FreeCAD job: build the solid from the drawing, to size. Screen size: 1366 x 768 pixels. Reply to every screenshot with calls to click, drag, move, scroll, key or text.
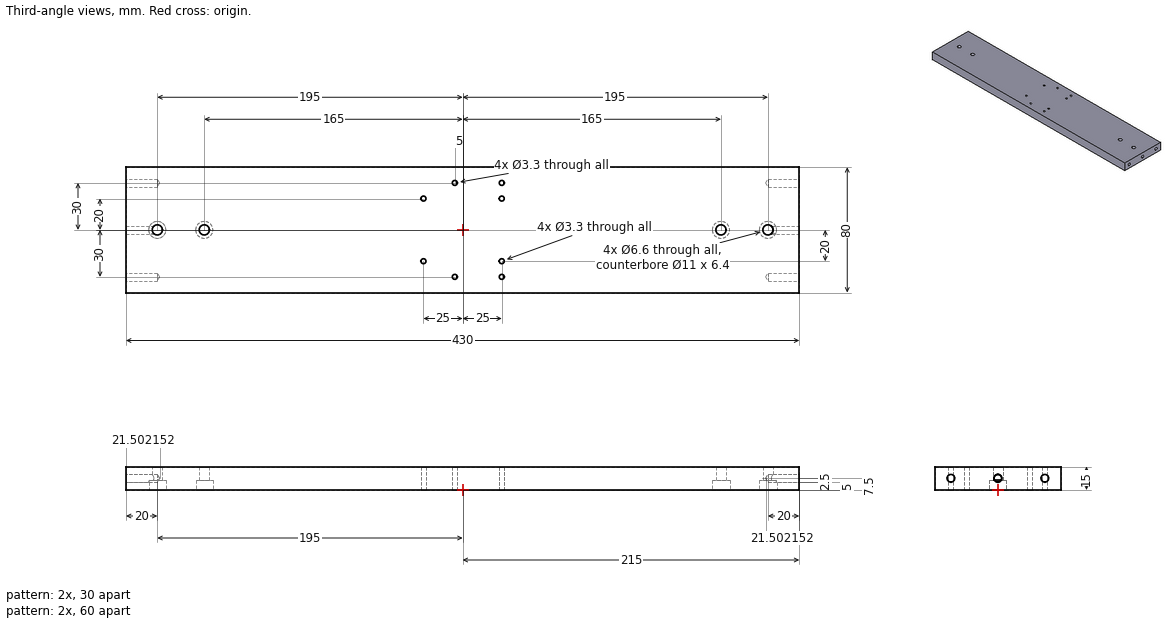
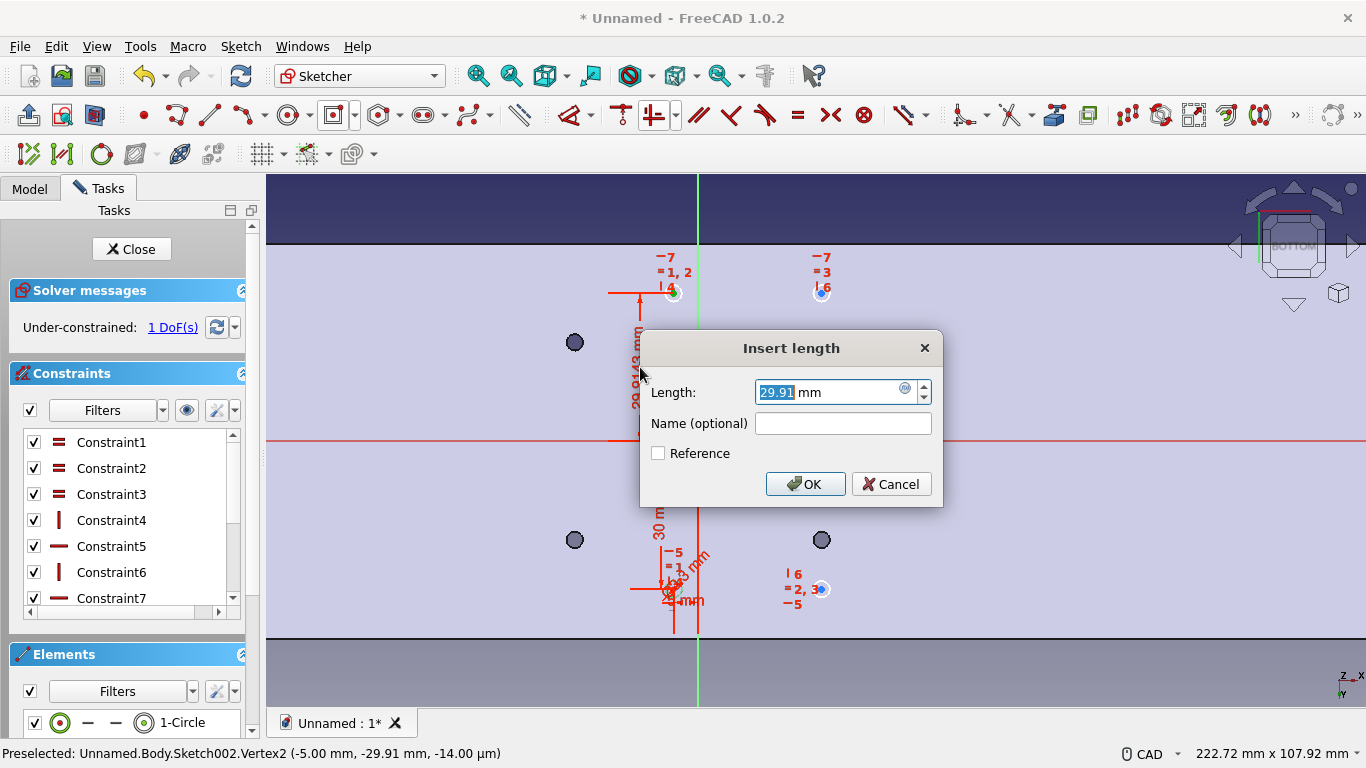
text(30)
key(Return)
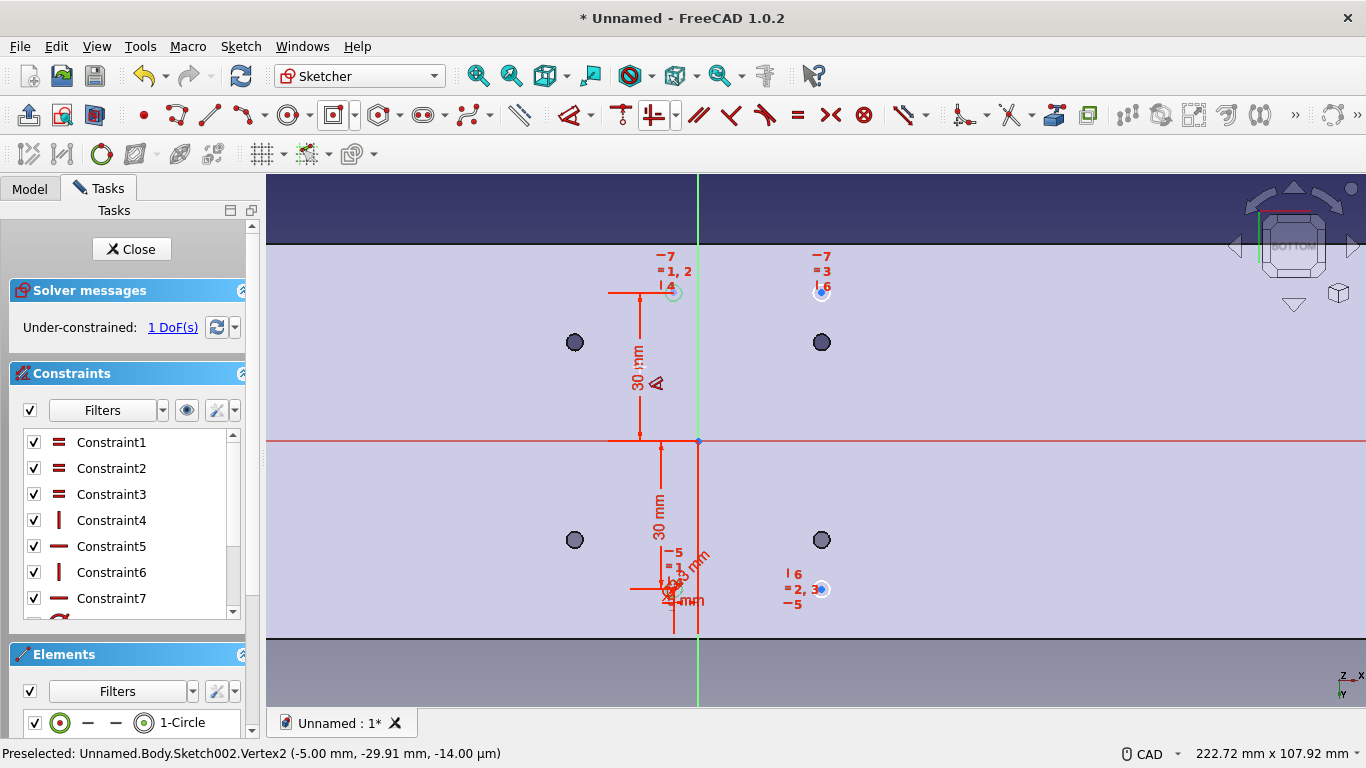
click(822, 589)
click(760, 623)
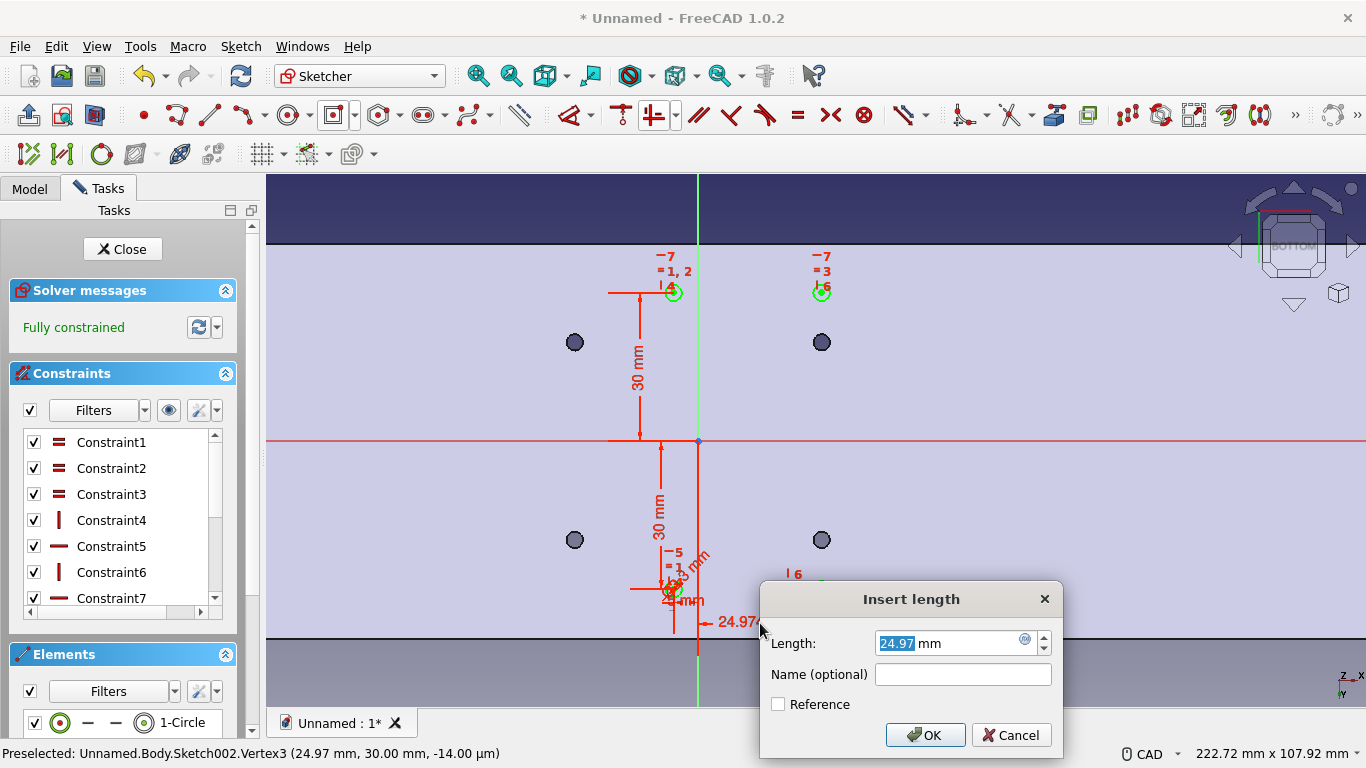
text(25)
key(Return)
key(Escape)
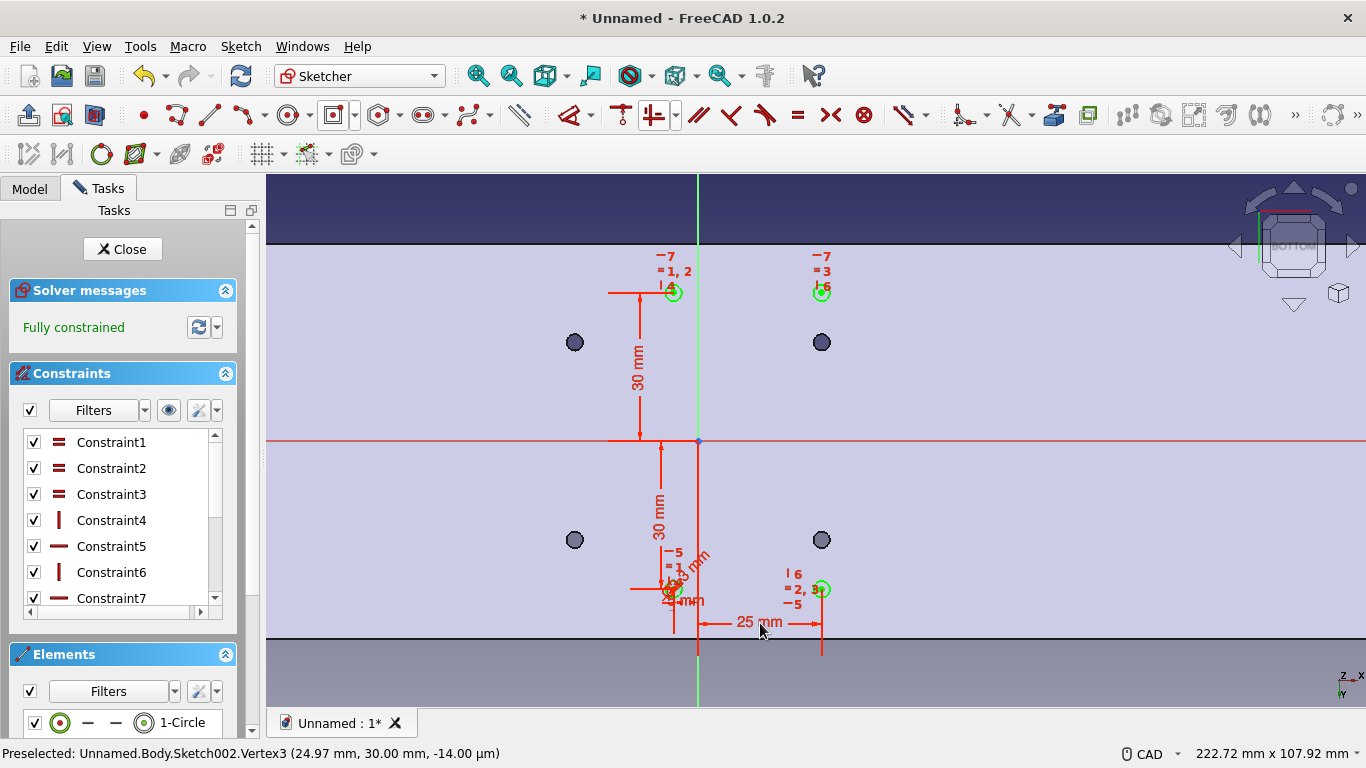
click(123, 249)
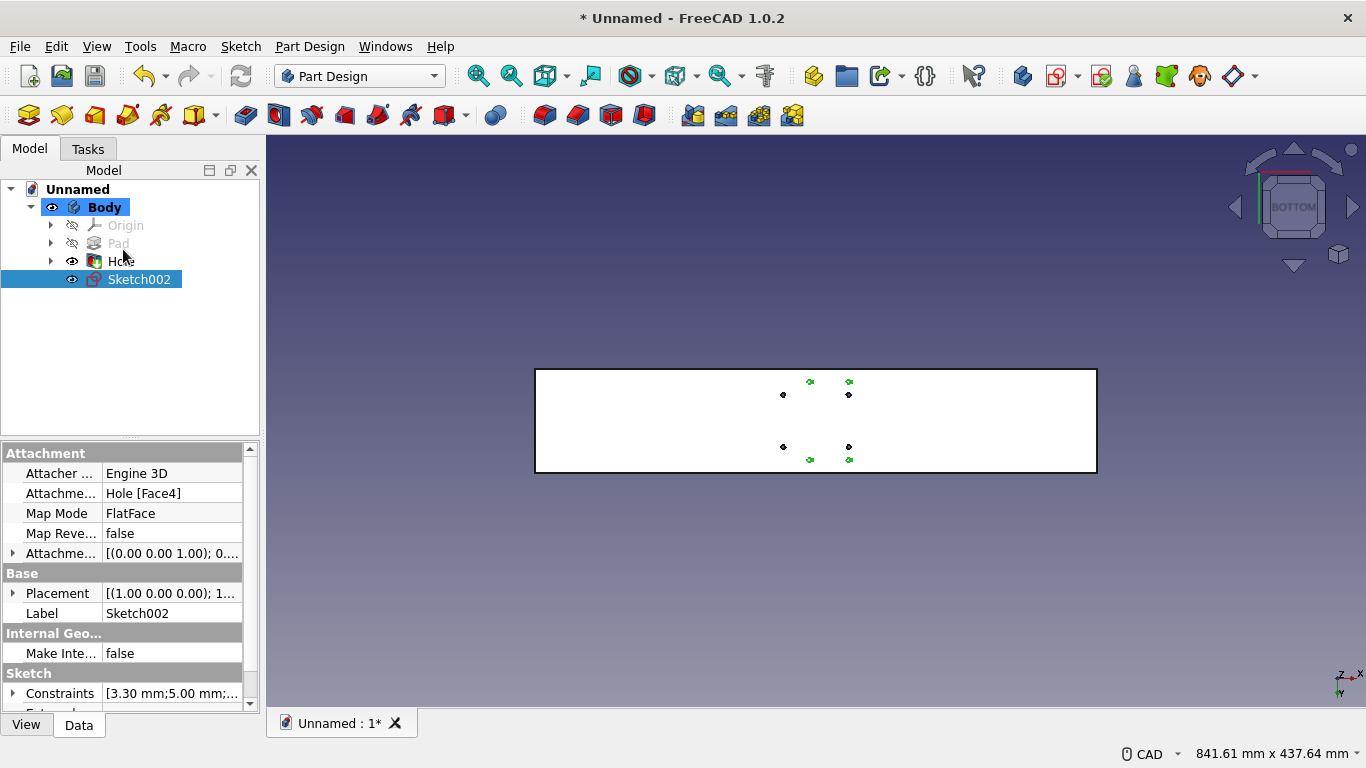
click(279, 116)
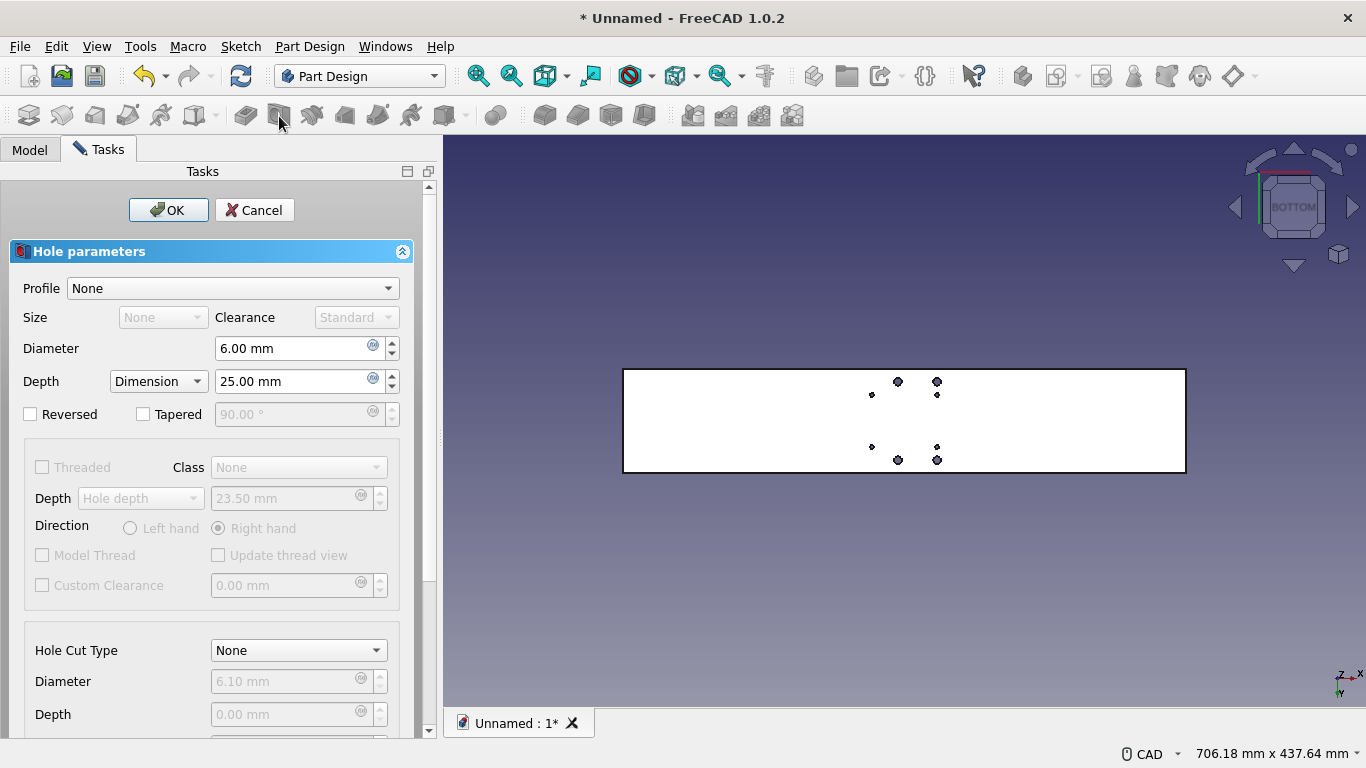
triple_click(300, 348)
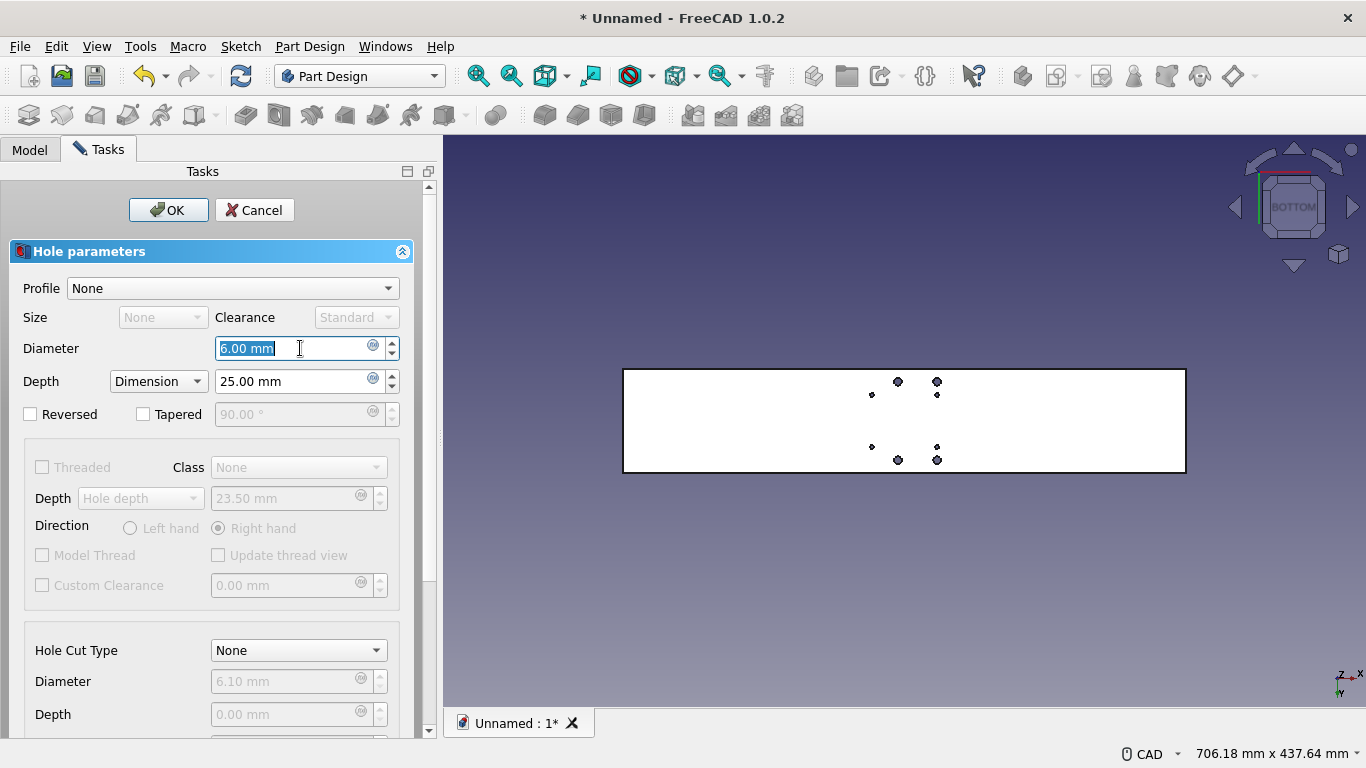
text(3.3)
key(Tab)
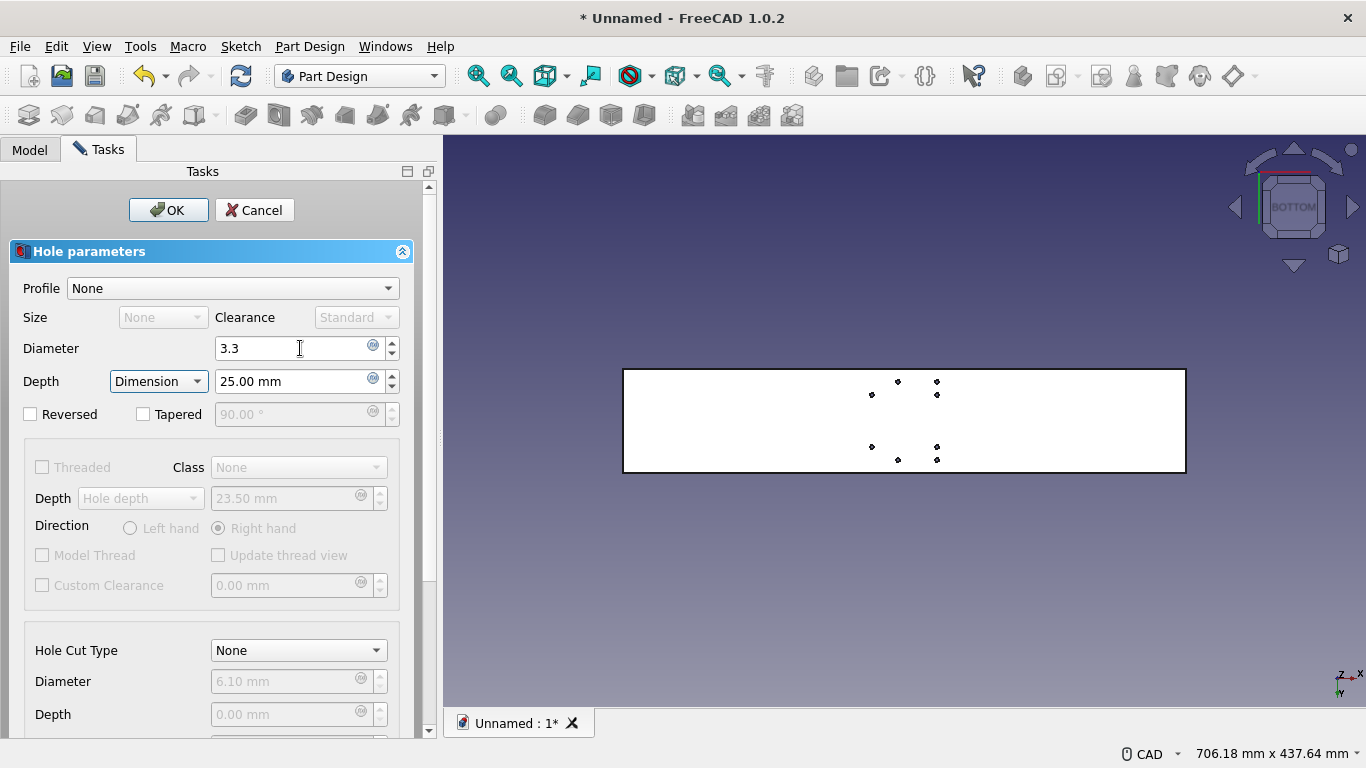
click(160, 382)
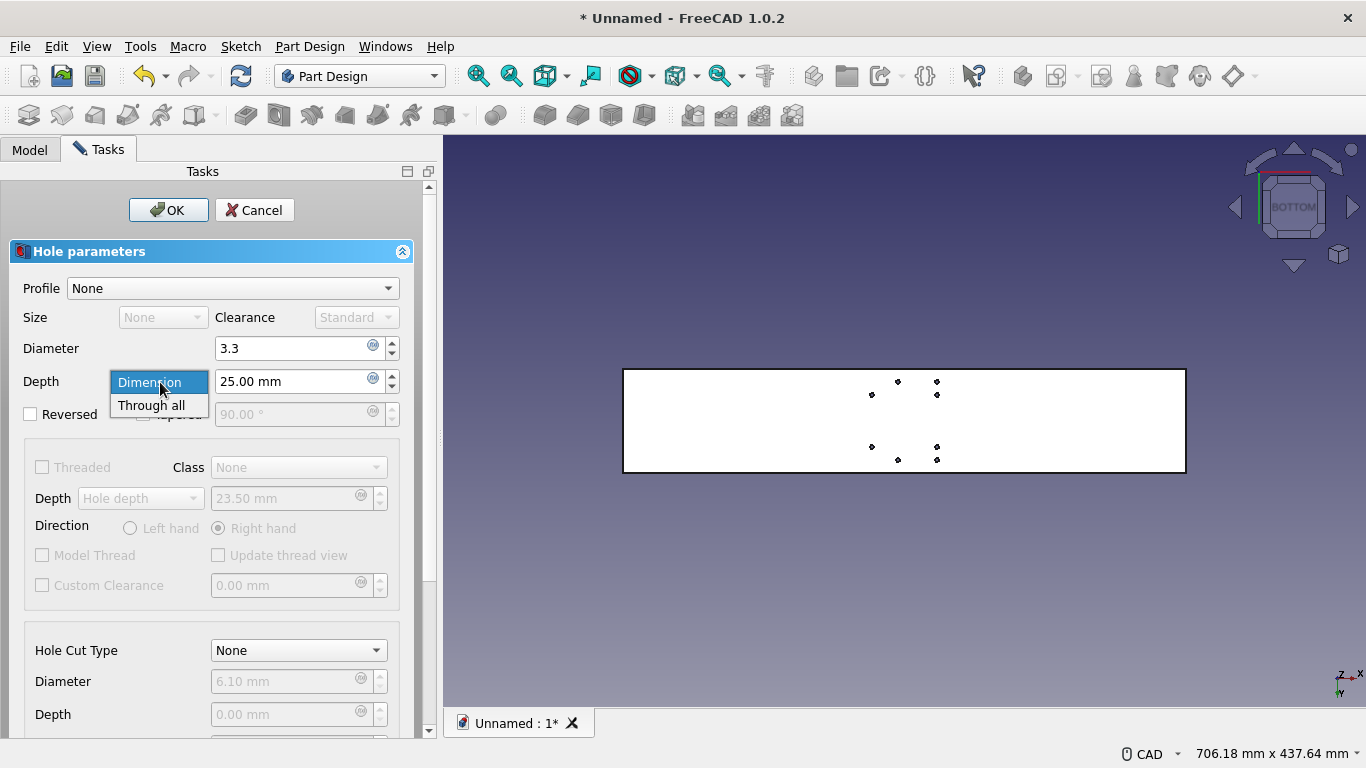
click(158, 406)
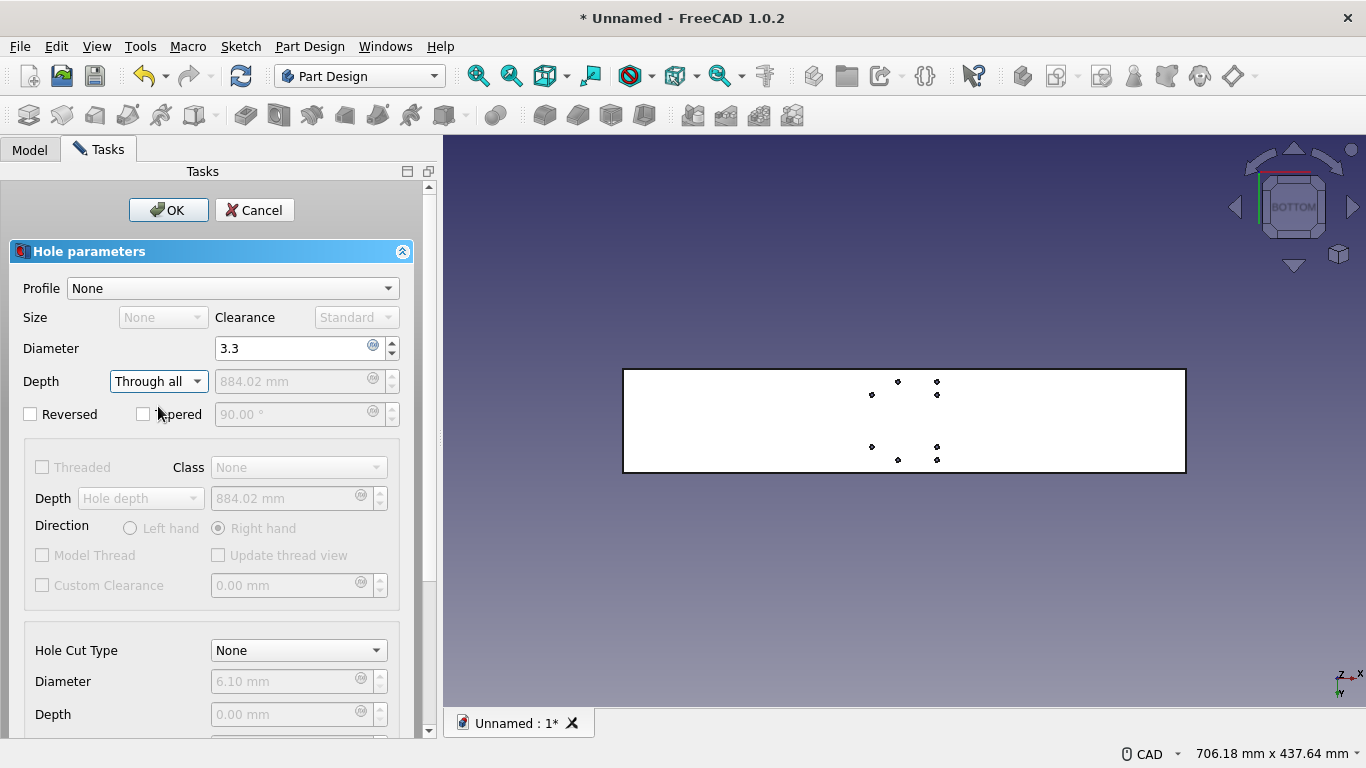
click(169, 210)